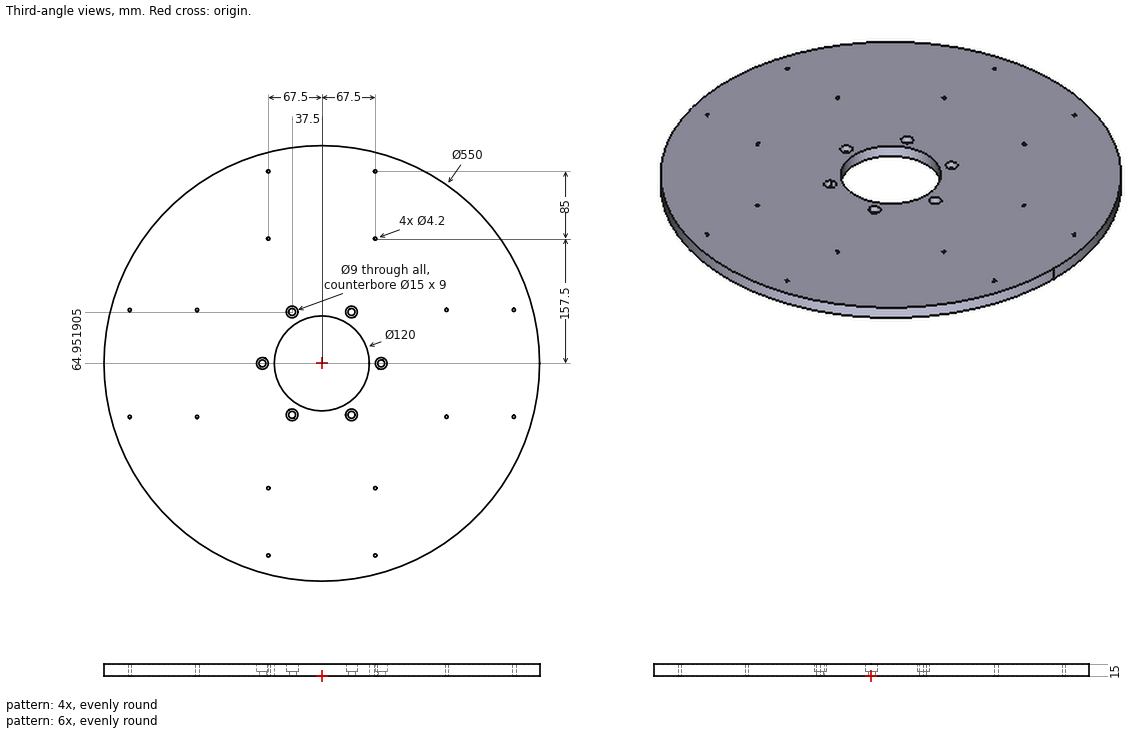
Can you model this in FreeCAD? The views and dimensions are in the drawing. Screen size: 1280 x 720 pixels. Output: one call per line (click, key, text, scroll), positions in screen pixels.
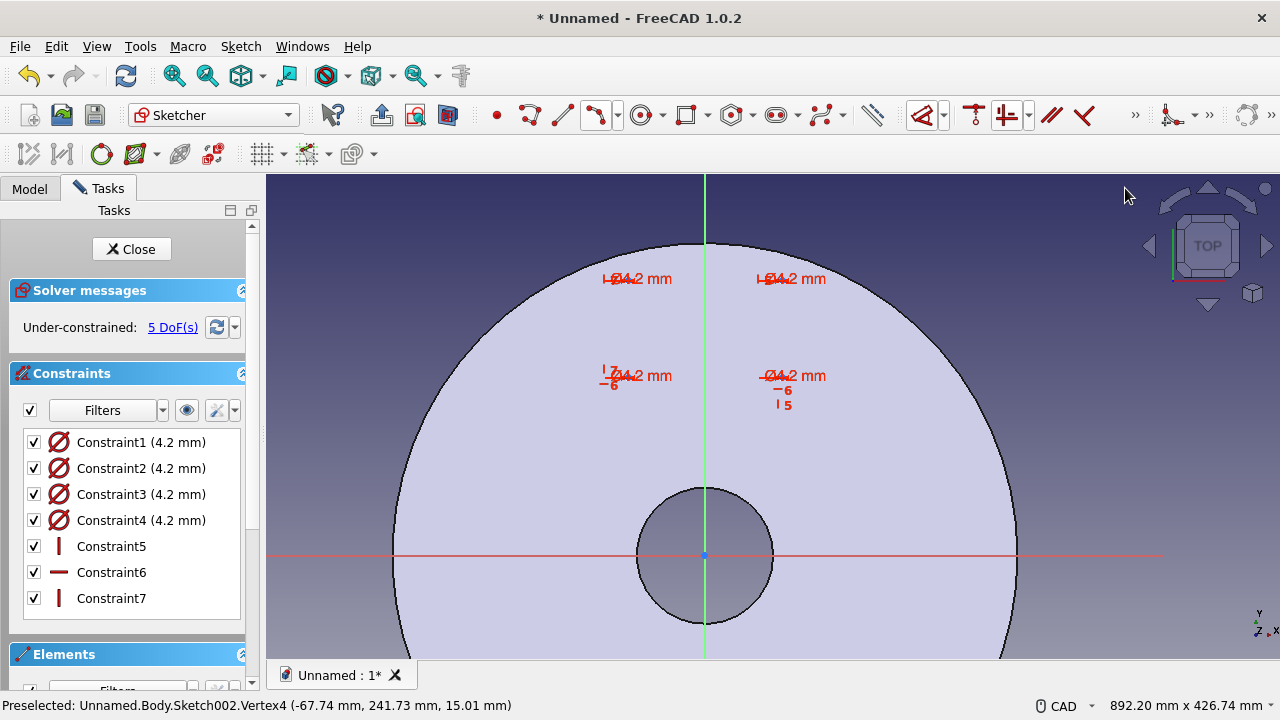
click(782, 281)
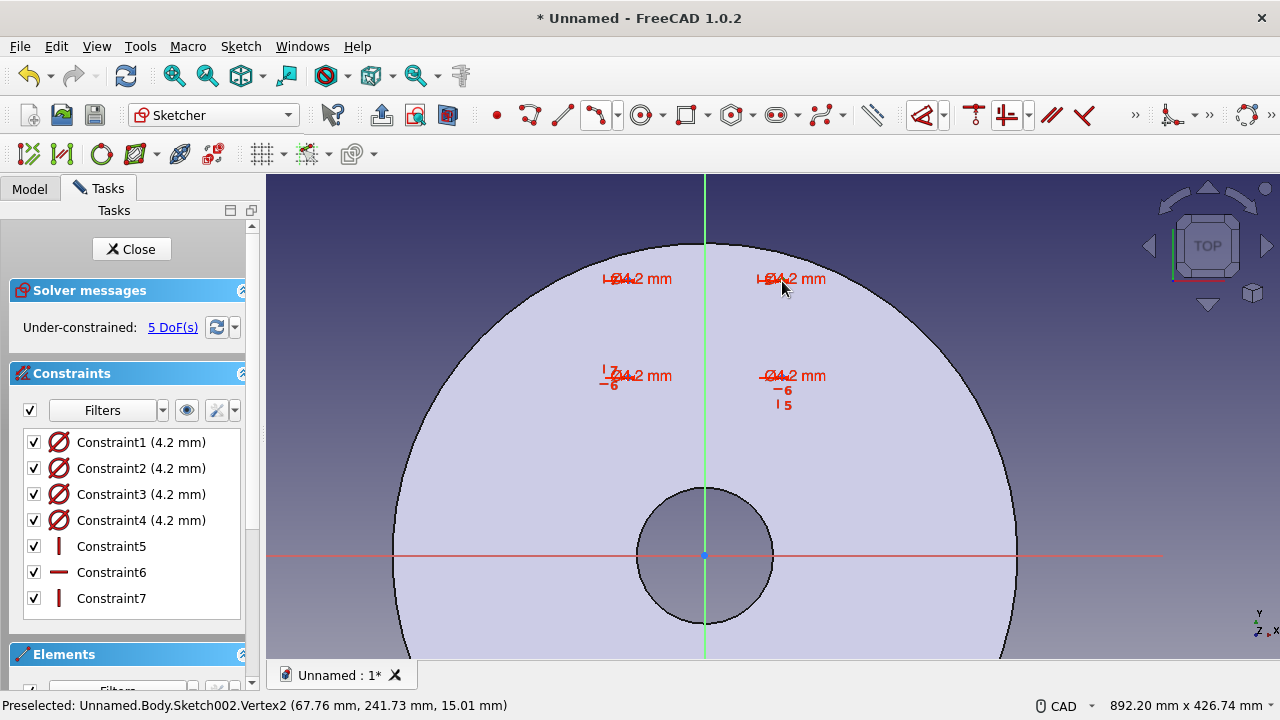
click(628, 281)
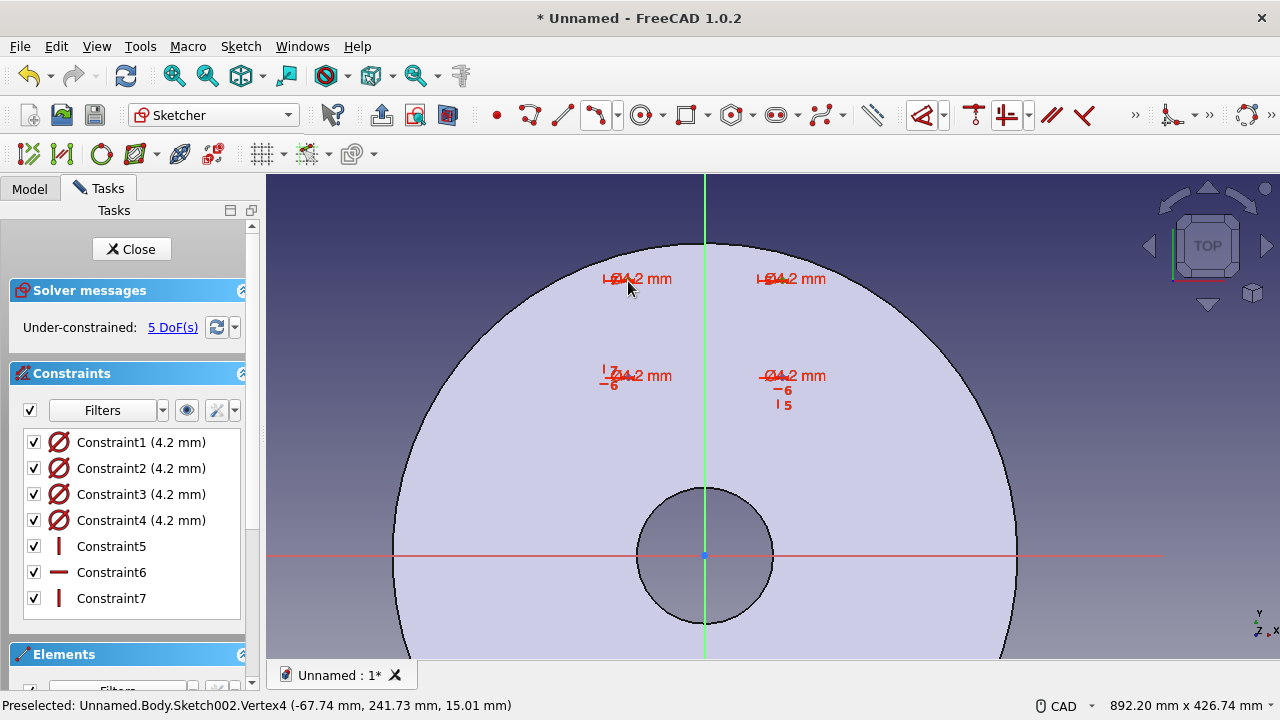
click(1028, 116)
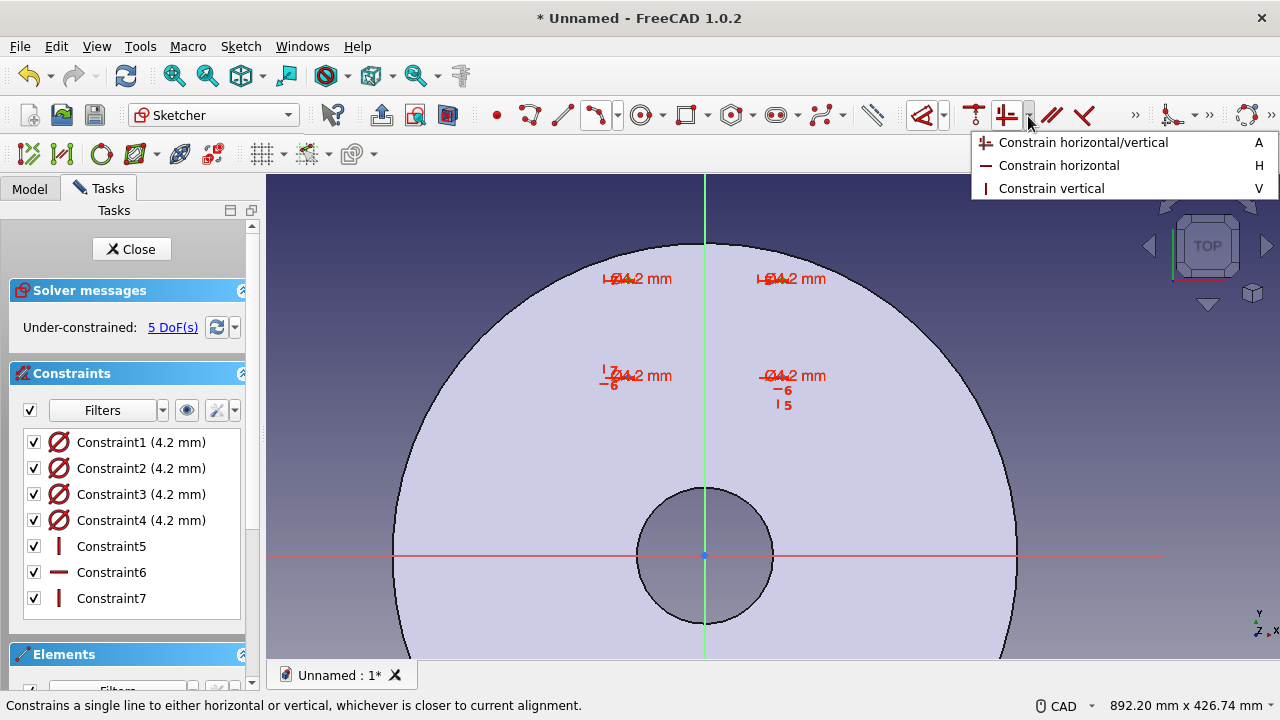
click(1125, 166)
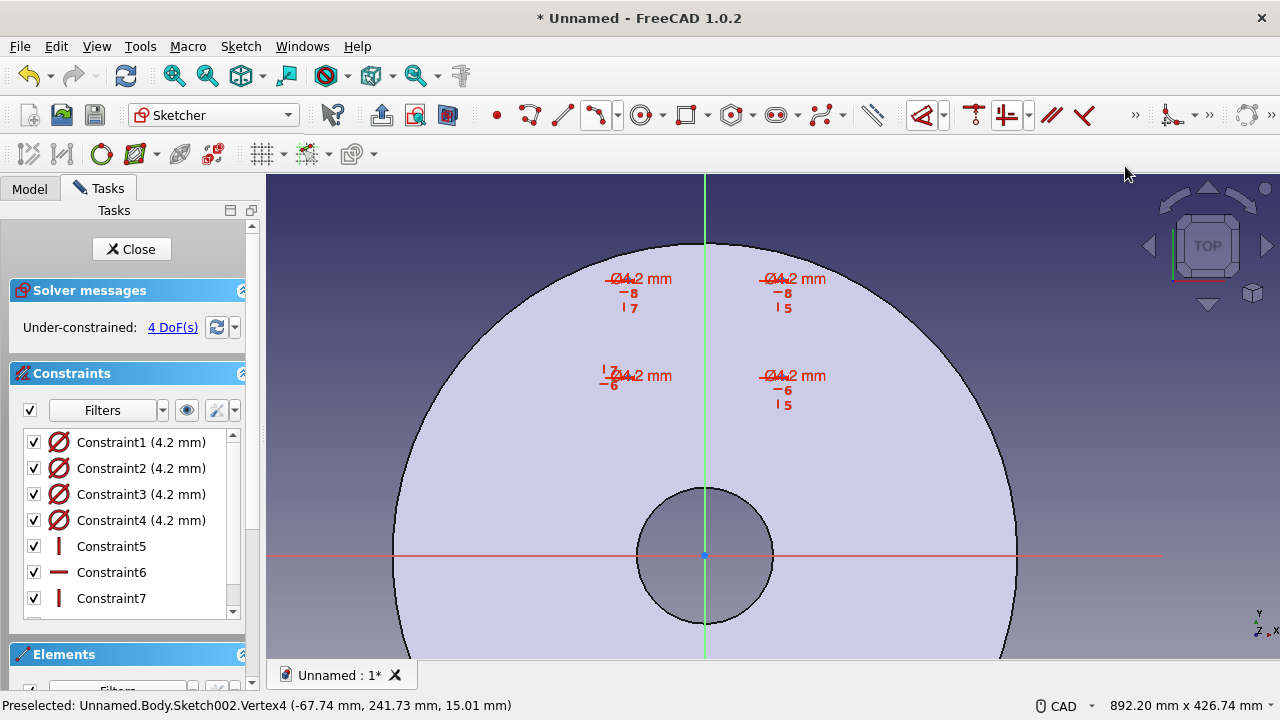
click(922, 116)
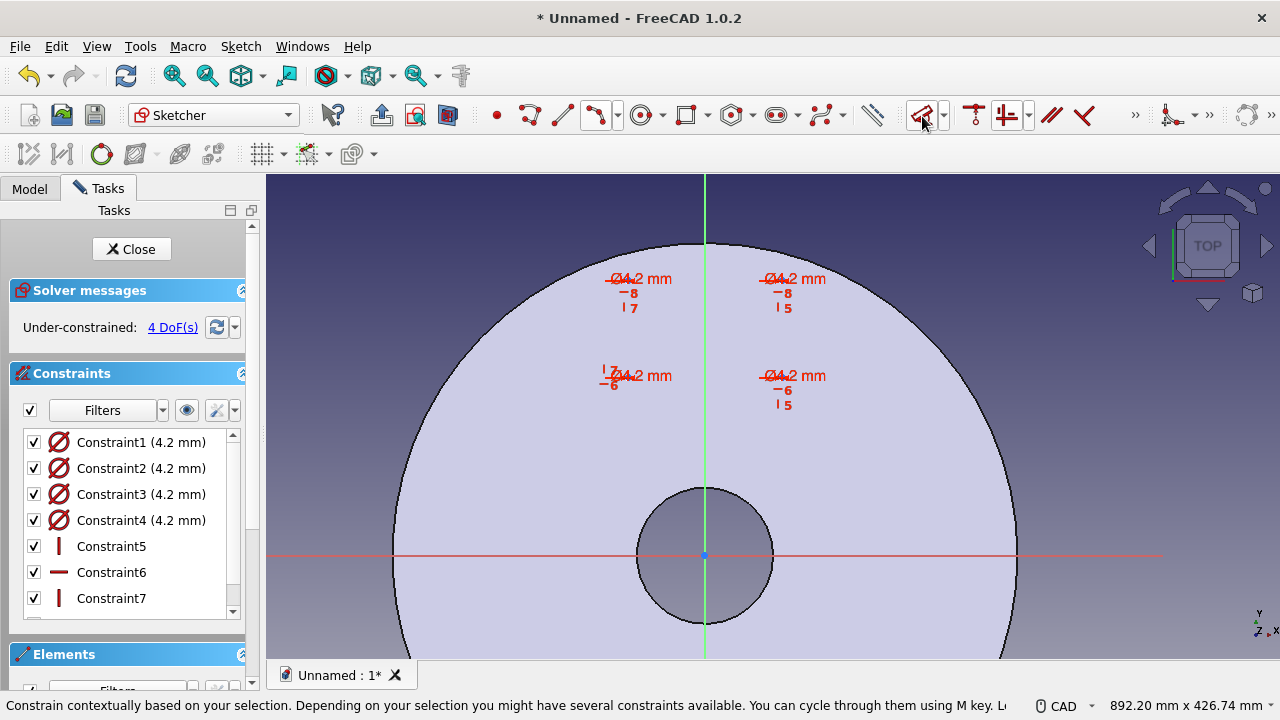
click(782, 378)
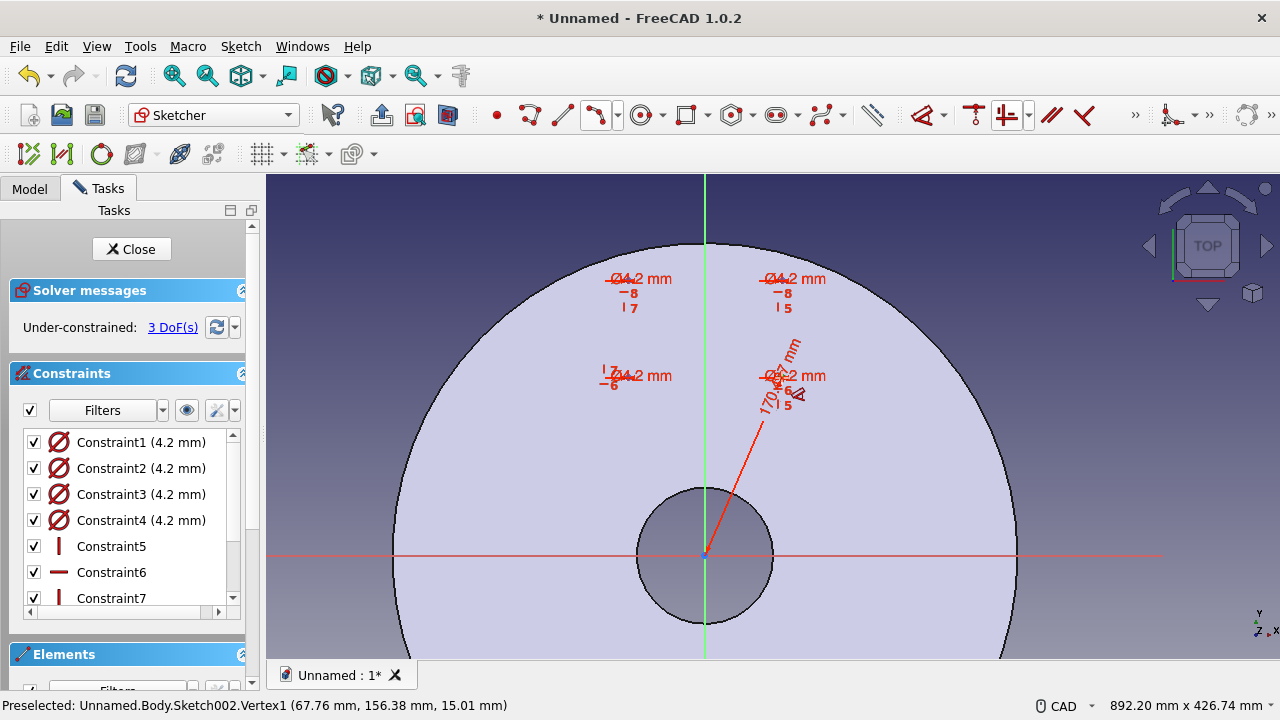
click(782, 281)
click(816, 329)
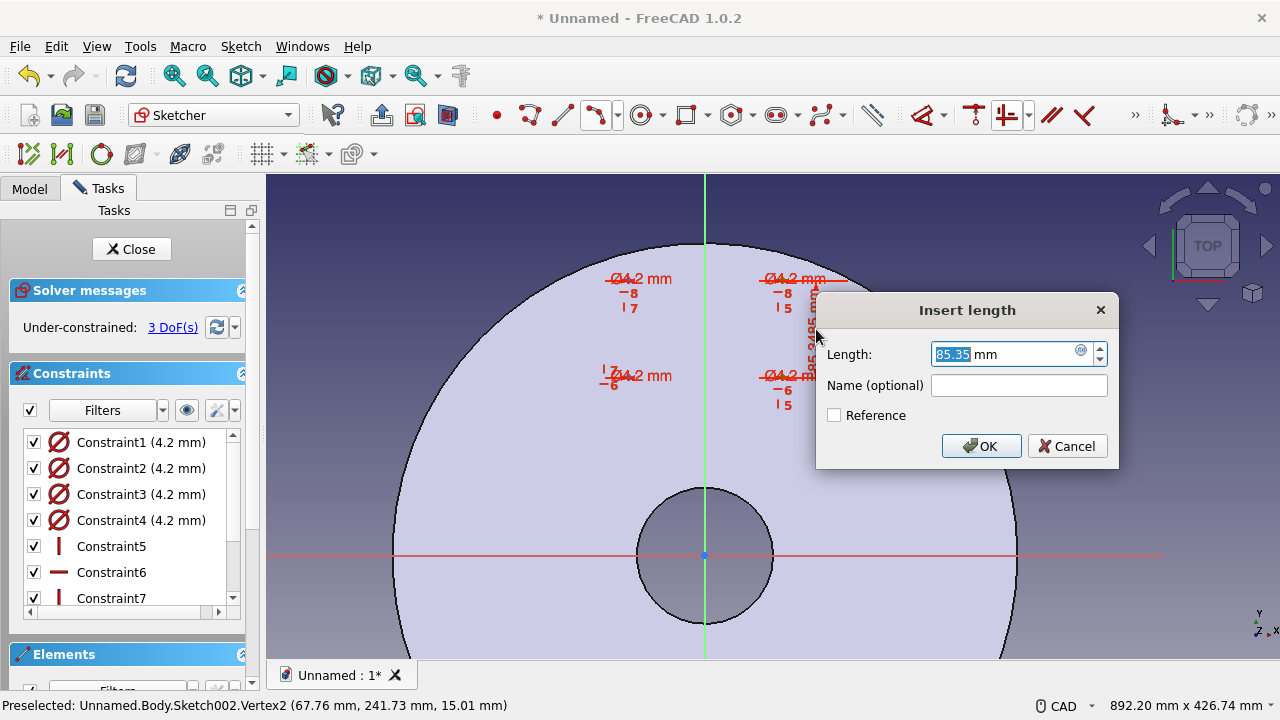
text(85)
key(Return)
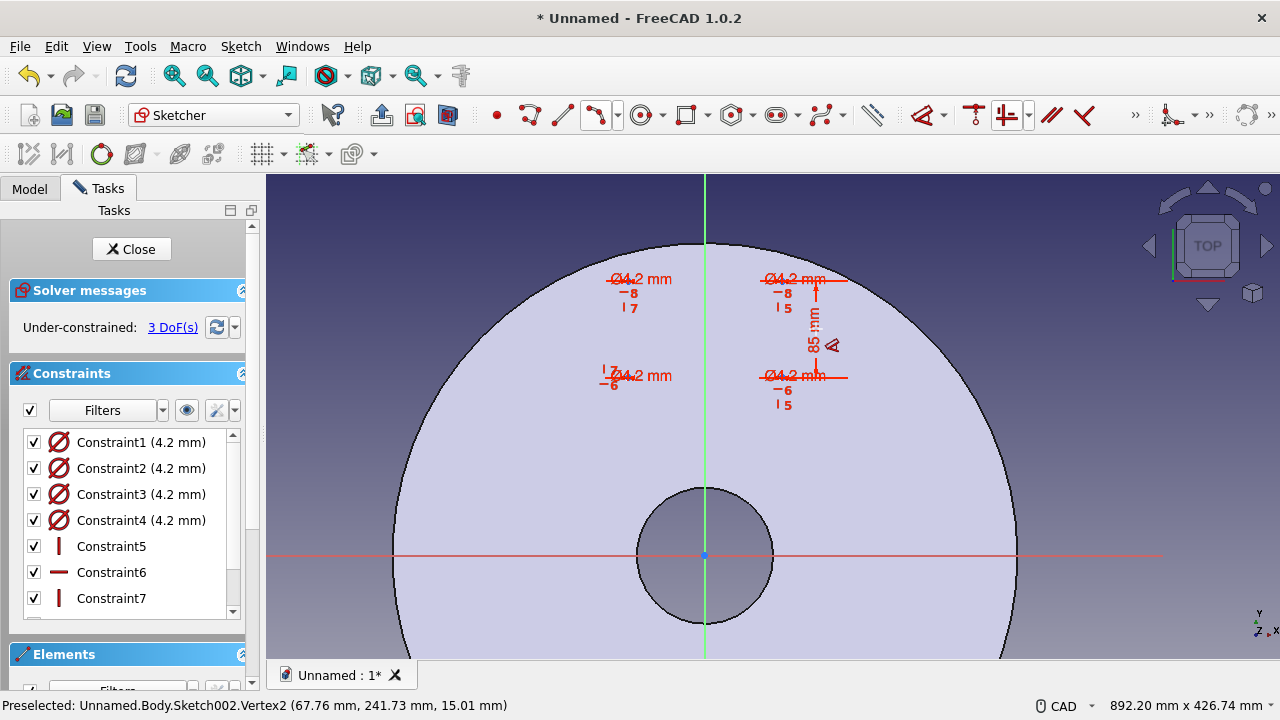
click(782, 378)
click(743, 590)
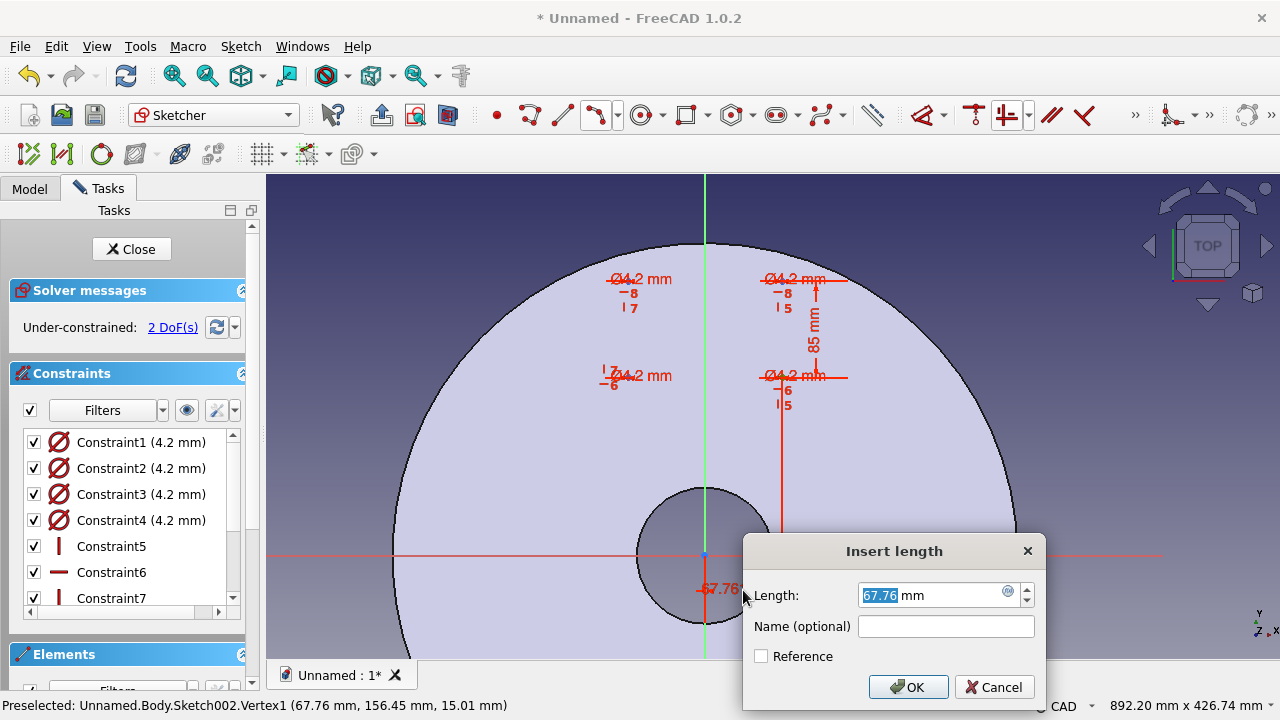
text(67.5)
key(Return)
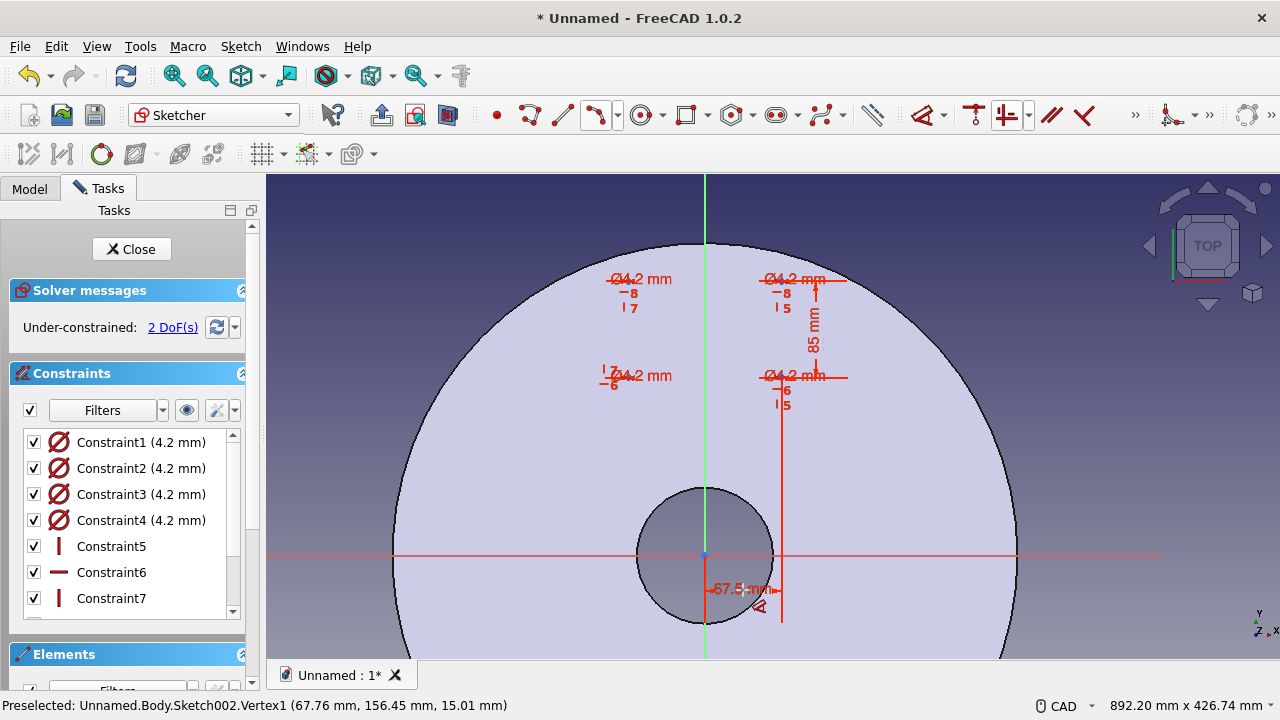
click(628, 378)
click(666, 590)